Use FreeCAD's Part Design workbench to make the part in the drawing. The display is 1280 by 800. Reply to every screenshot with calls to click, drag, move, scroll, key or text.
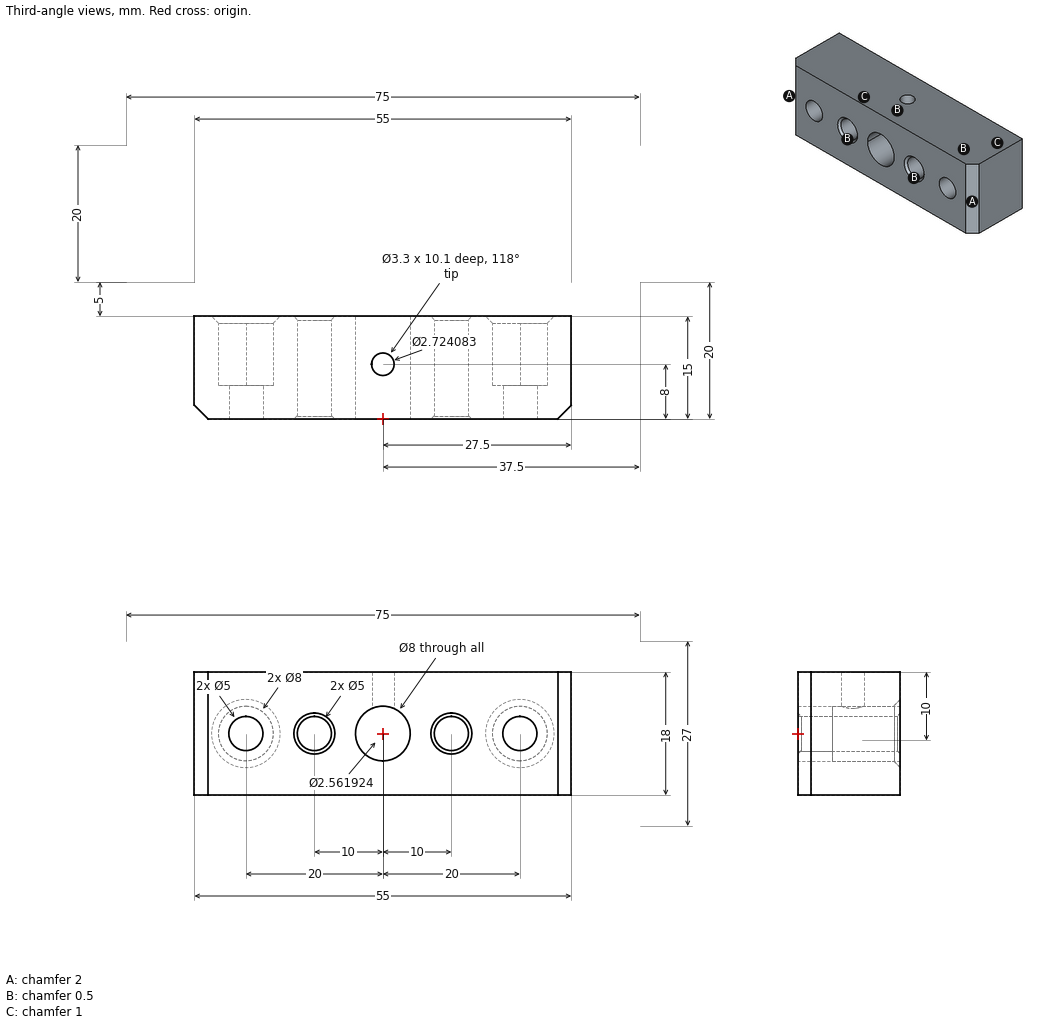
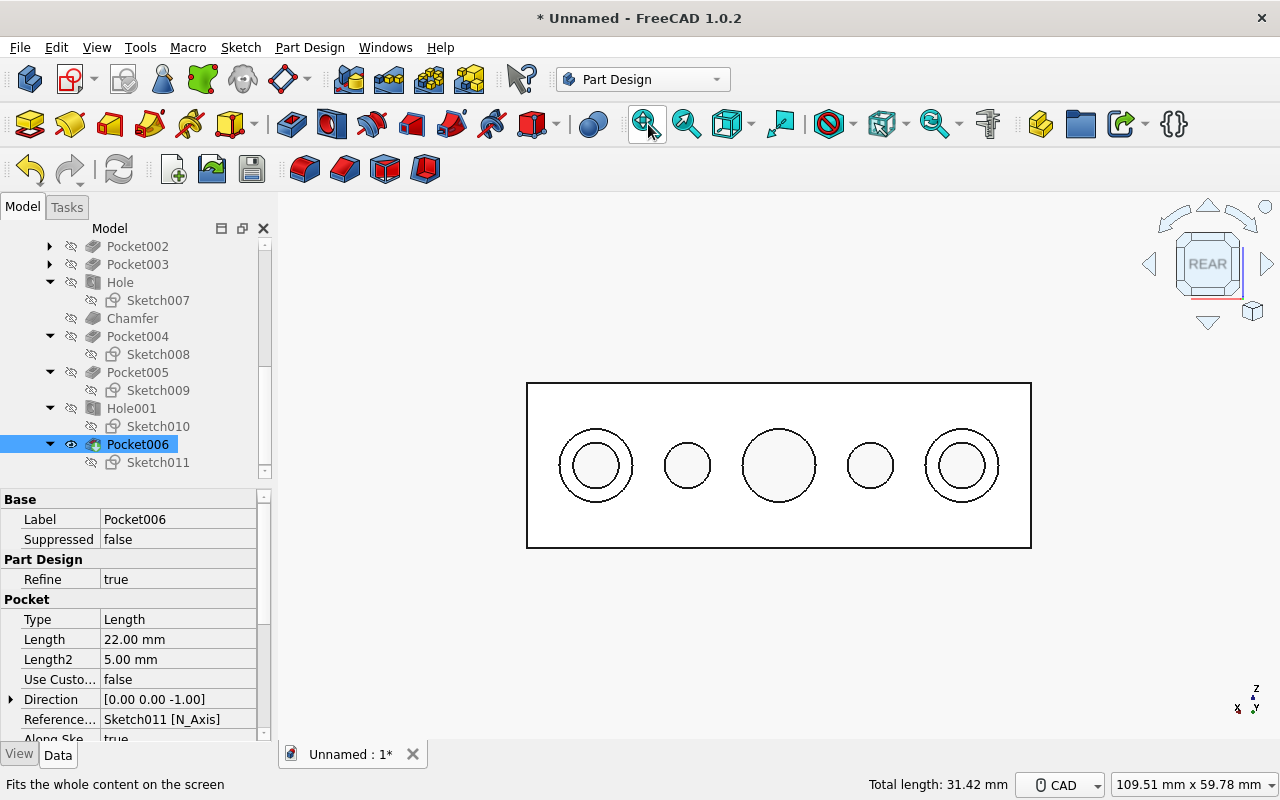
click(710, 465, ctrl)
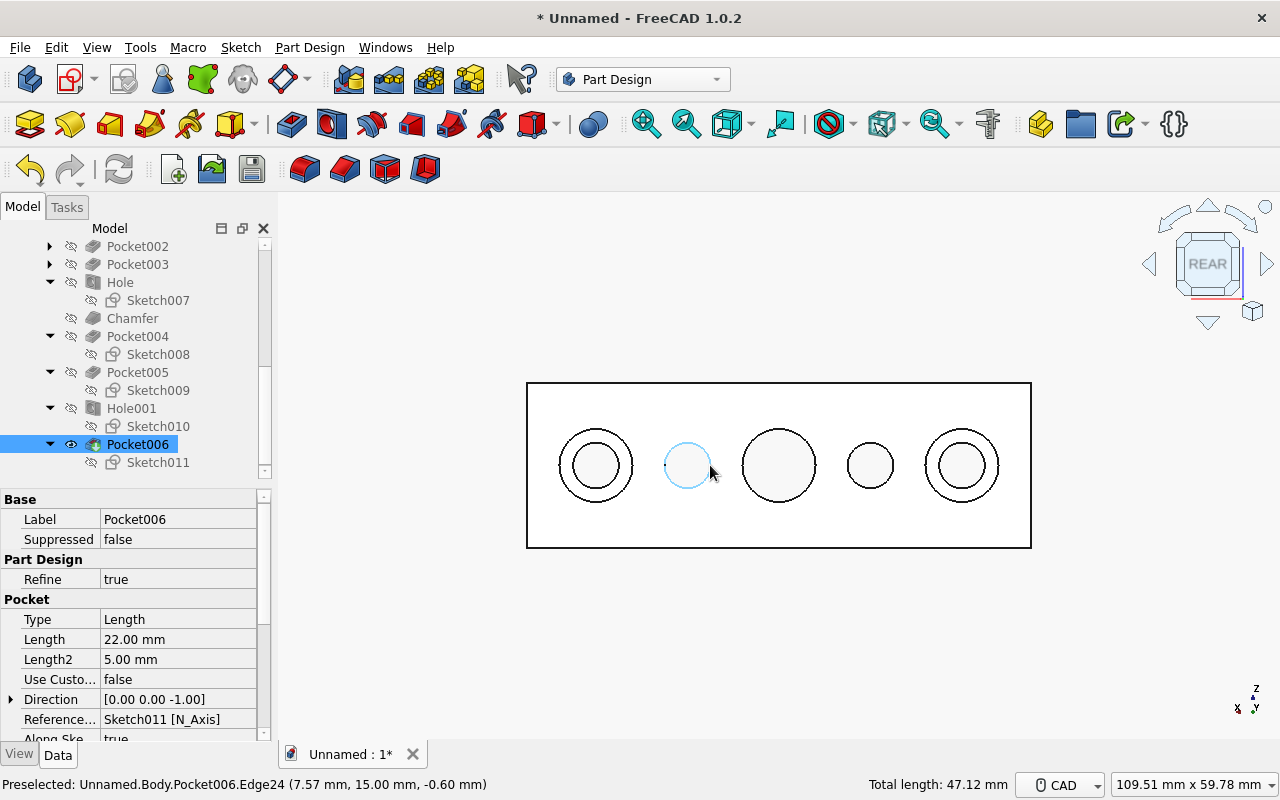
click(893, 465, ctrl)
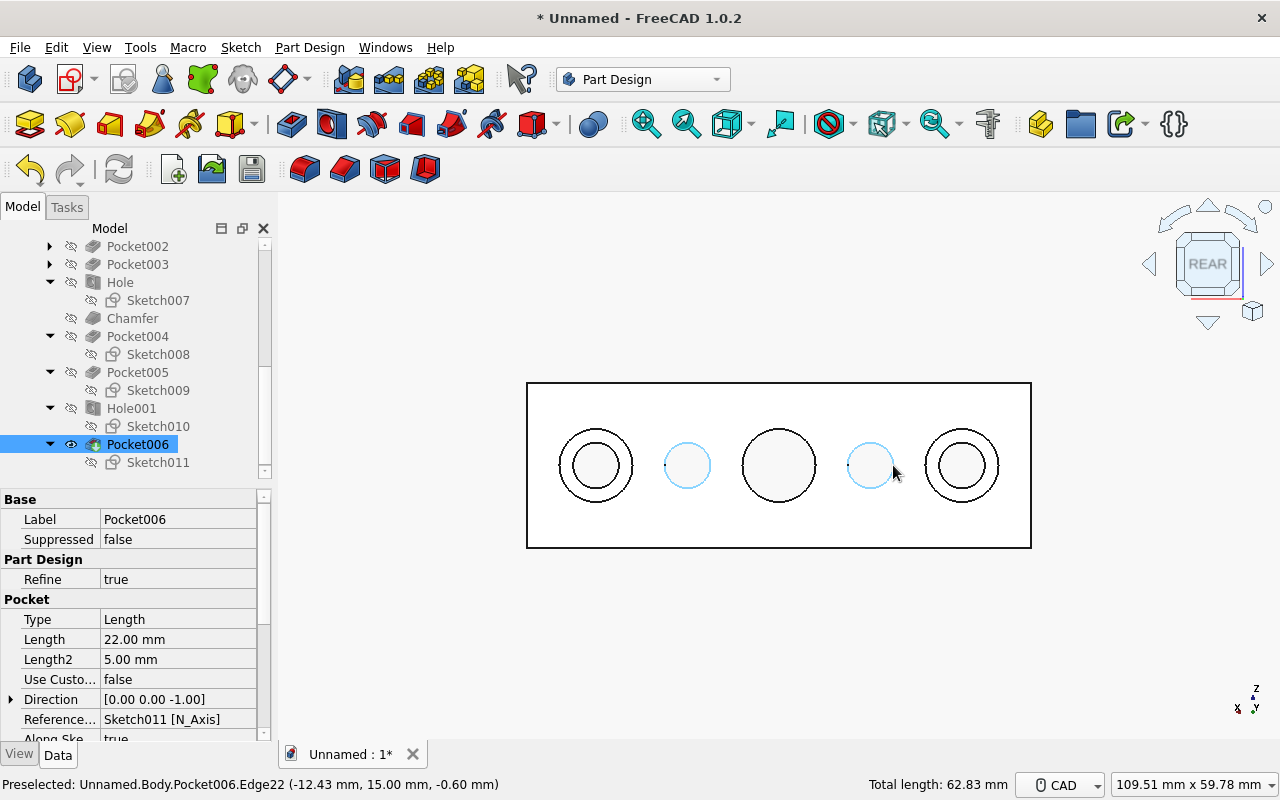
click(346, 170)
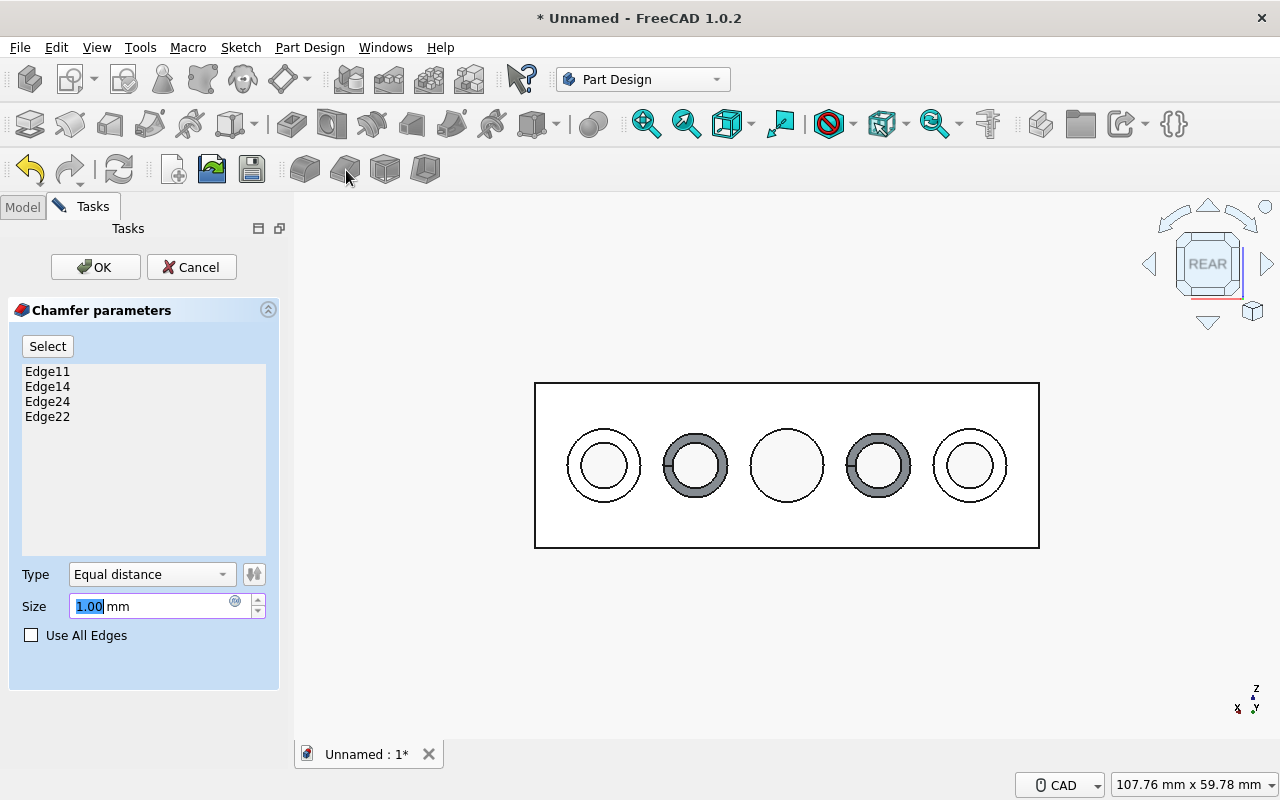
text(0.5)
key(Tab)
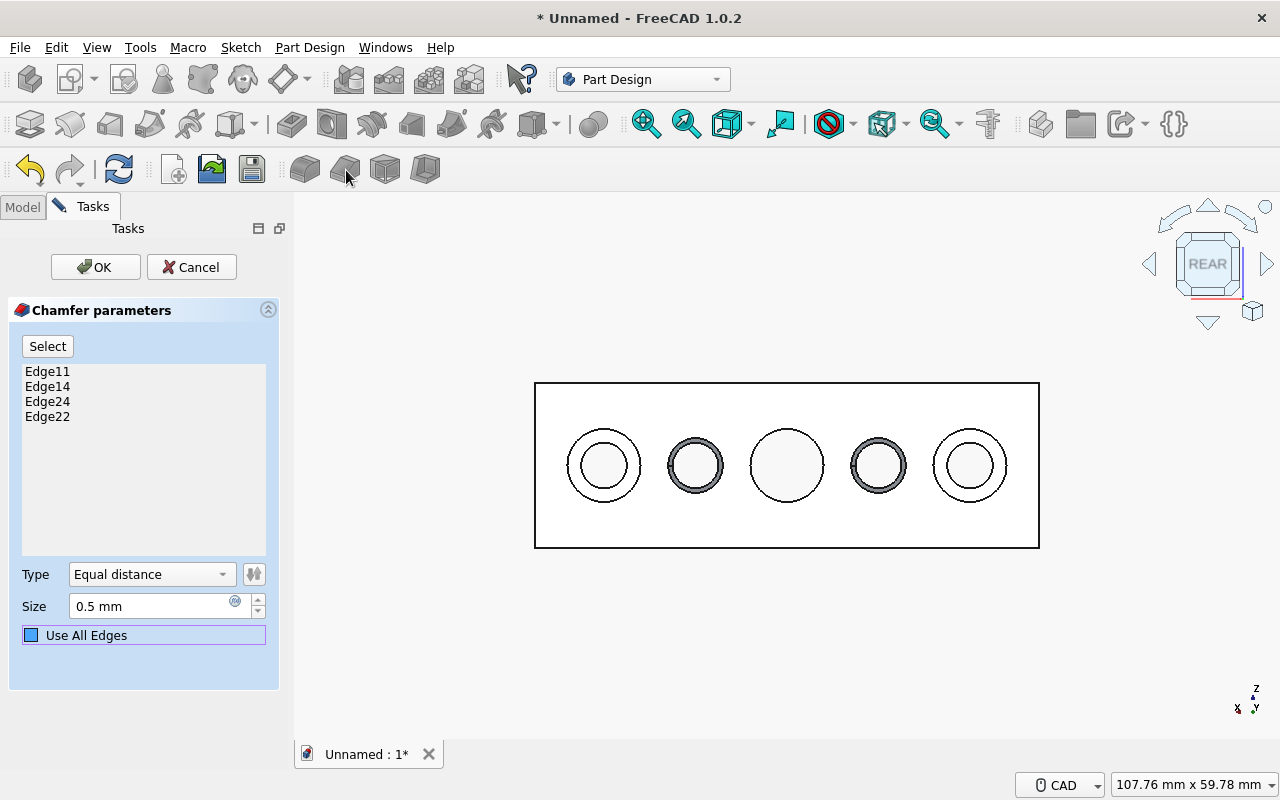
click(96, 267)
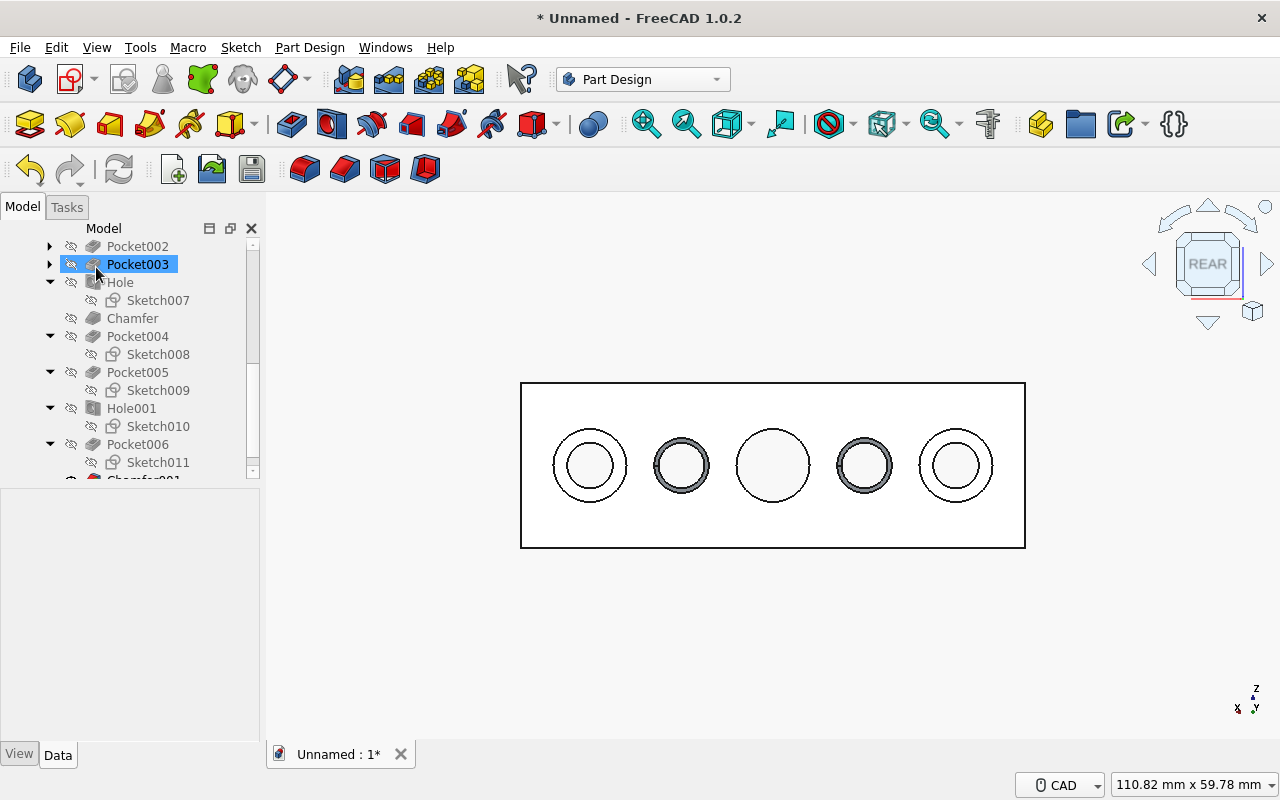
click(986, 443)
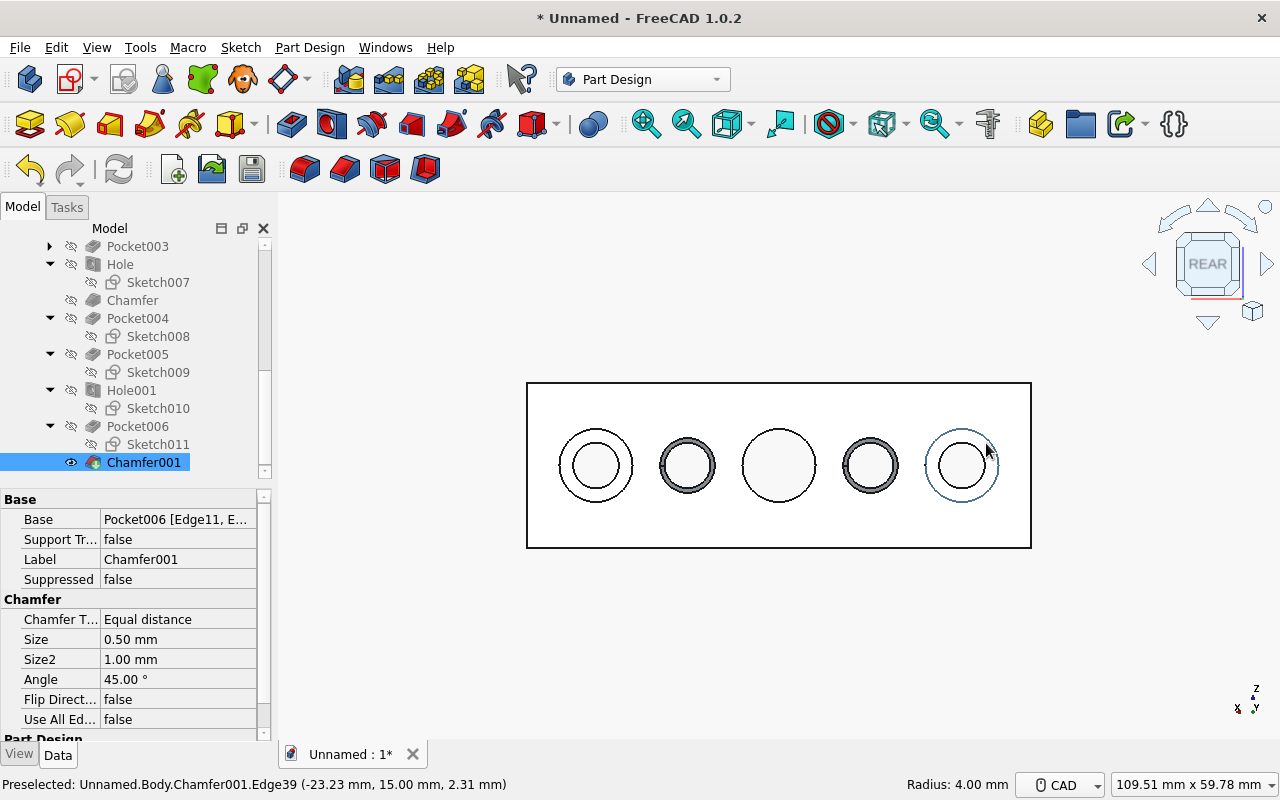
click(626, 443, ctrl)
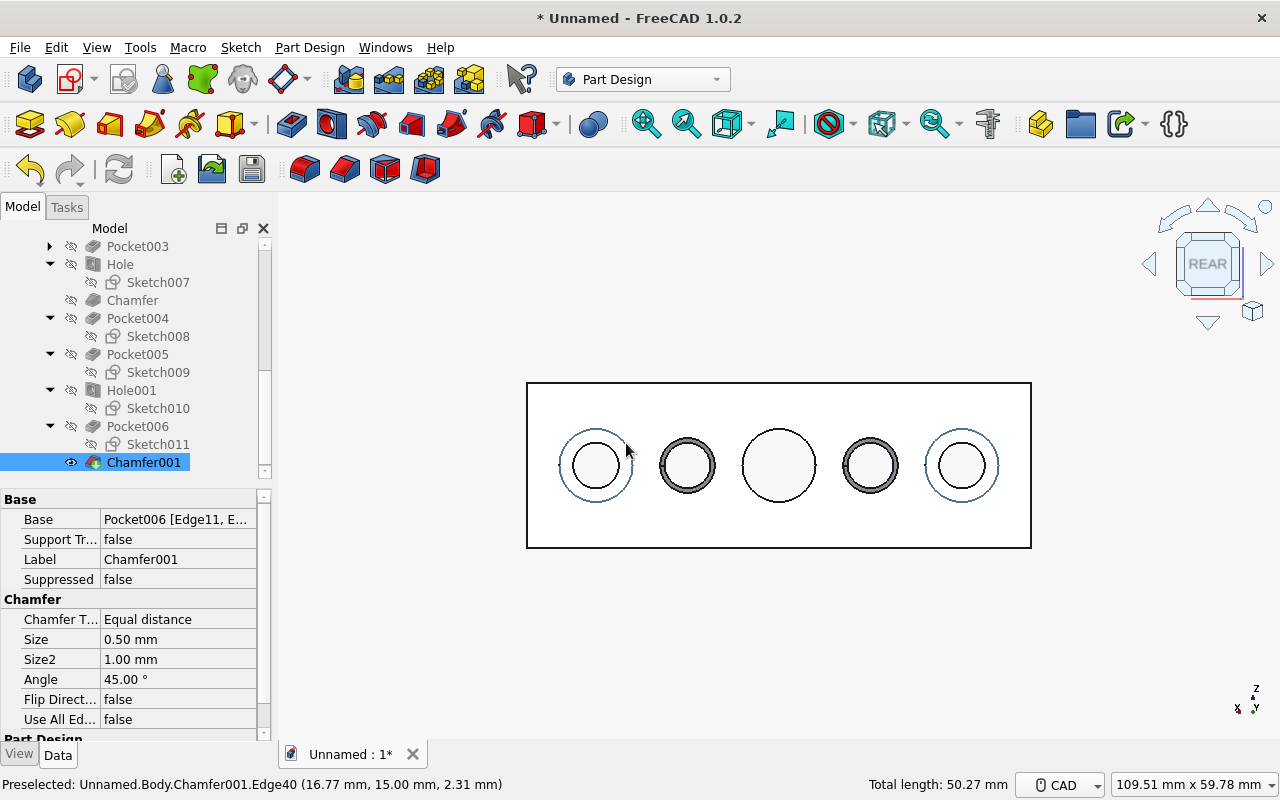
click(346, 170)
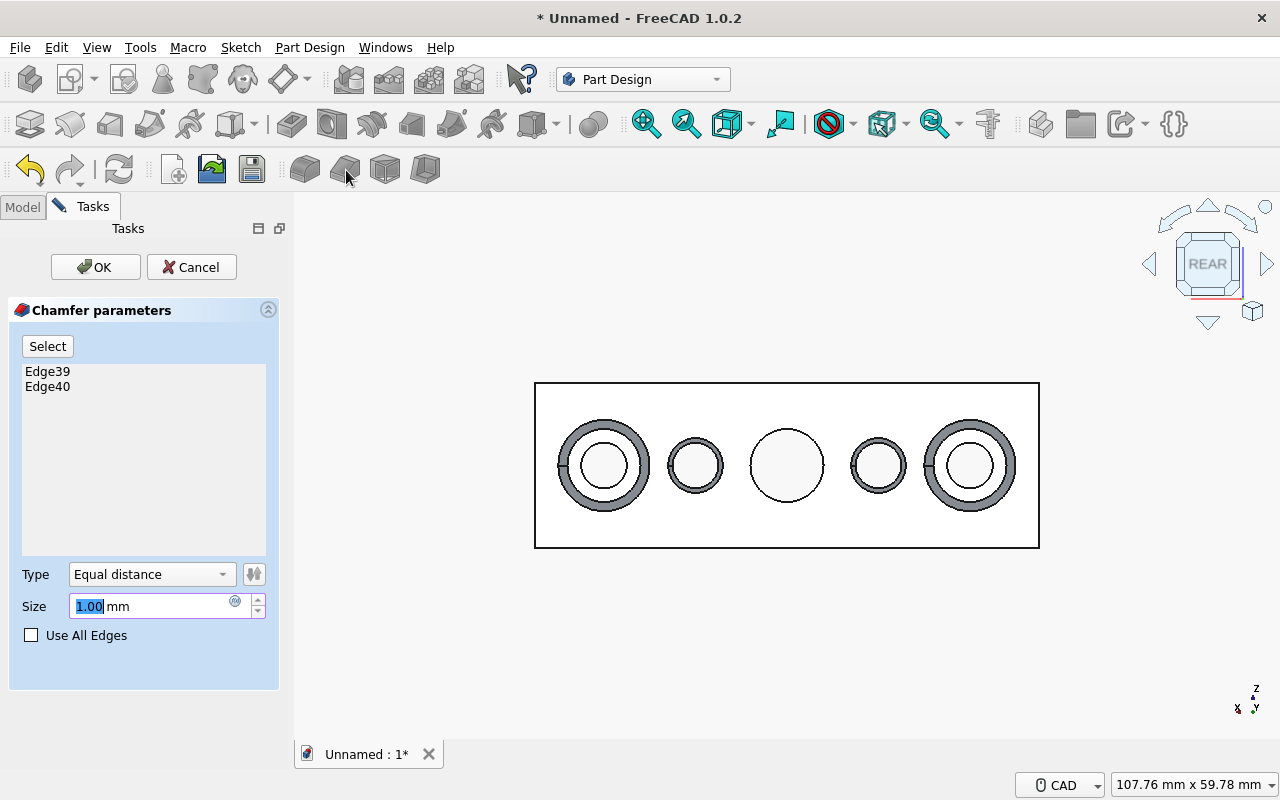
text(1)
key(Tab)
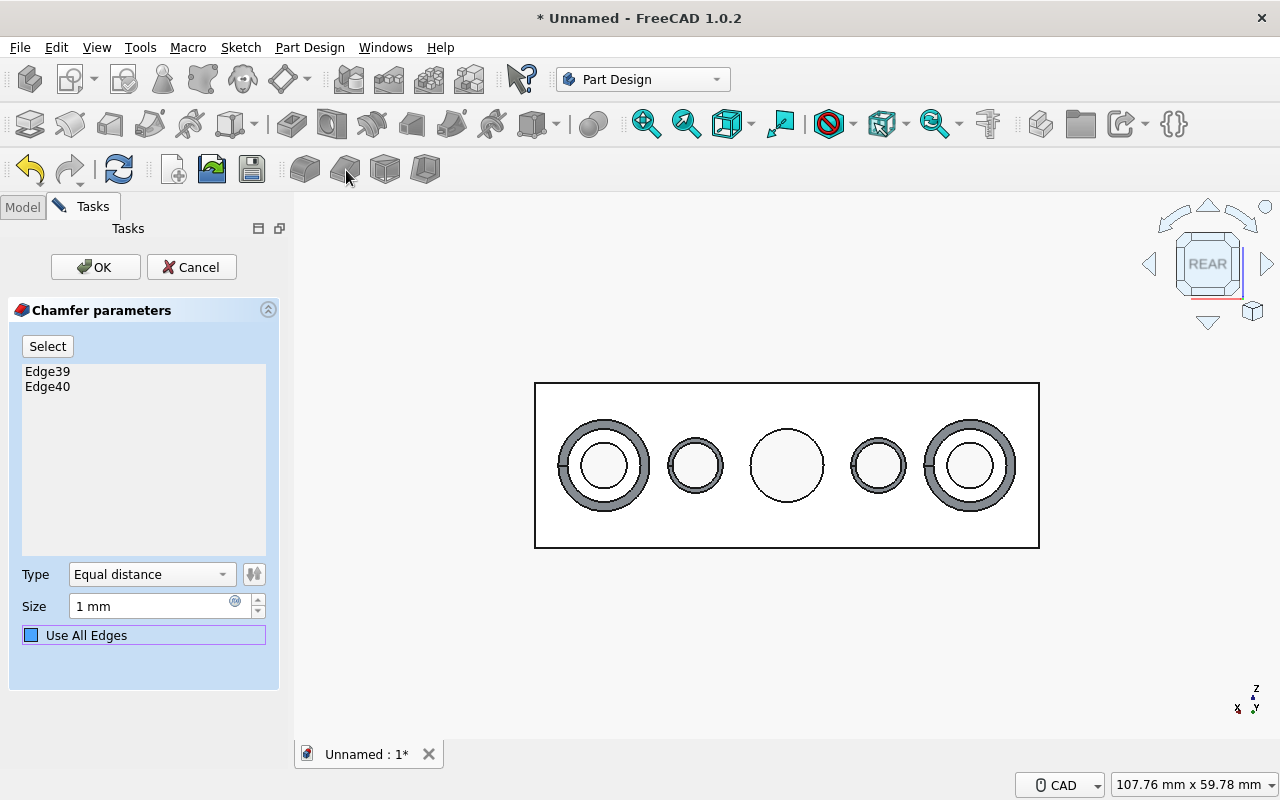
click(96, 267)